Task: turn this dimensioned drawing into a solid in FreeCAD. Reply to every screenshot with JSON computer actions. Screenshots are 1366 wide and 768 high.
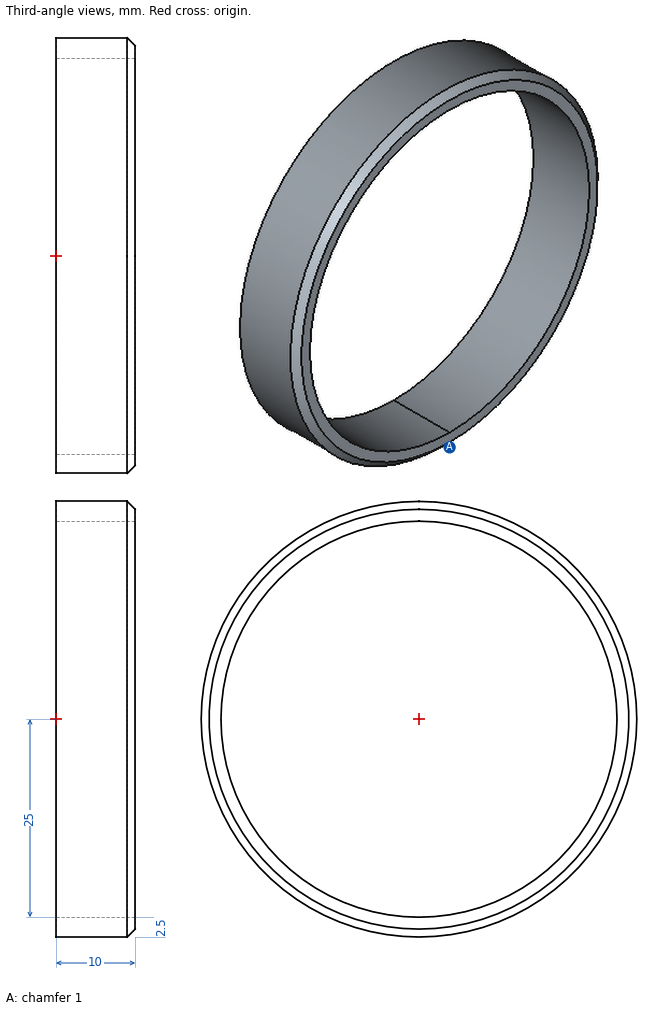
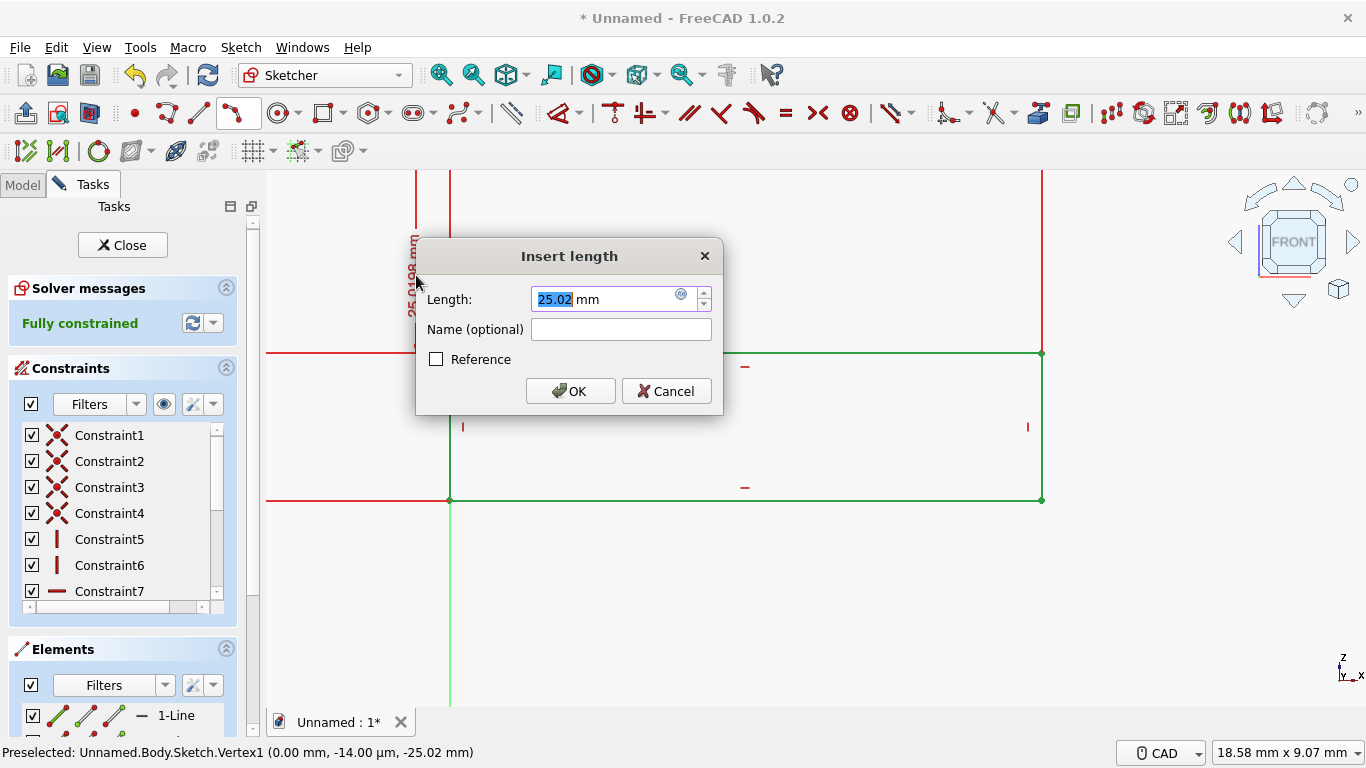
{"action": "type", "text": "25"}
{"action": "key", "text": "Return"}
{"action": "key", "text": "Escape"}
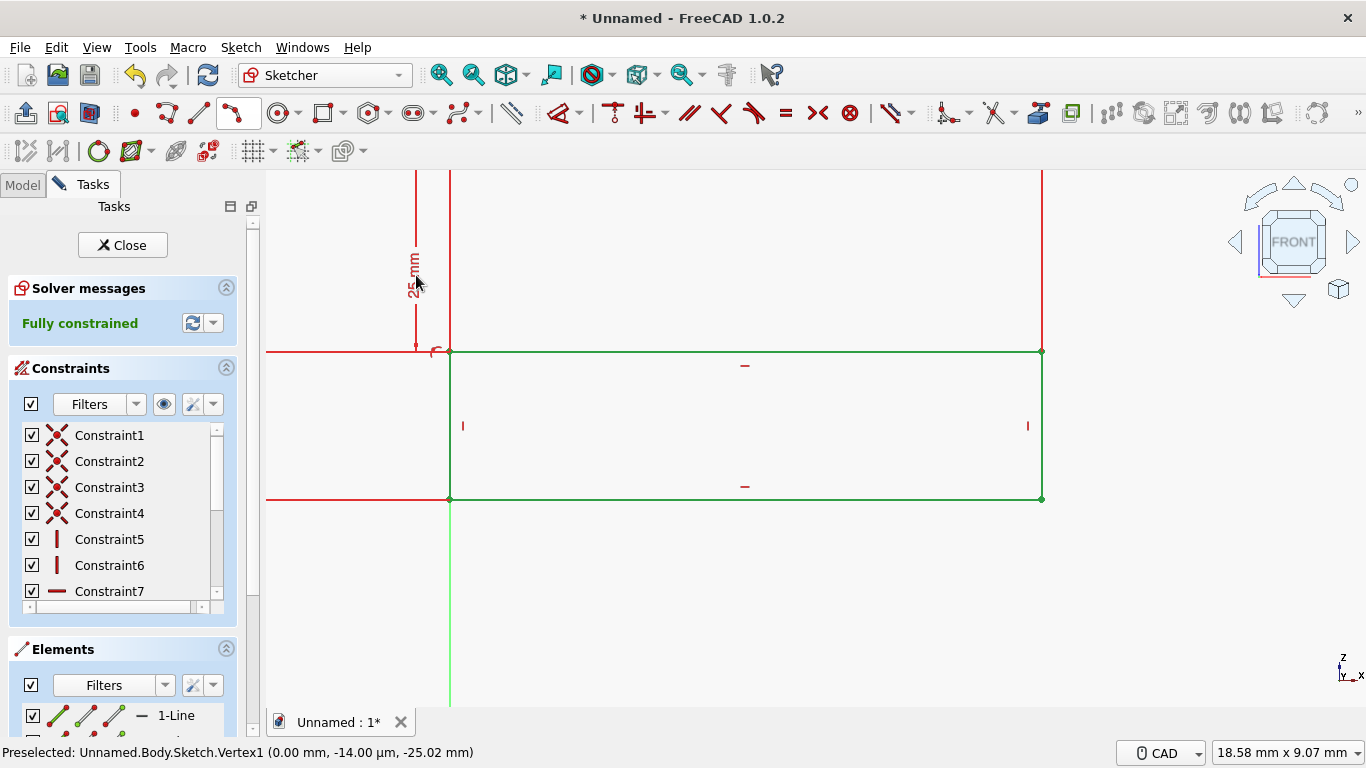
{"action": "left_click", "coordinate": [123, 245]}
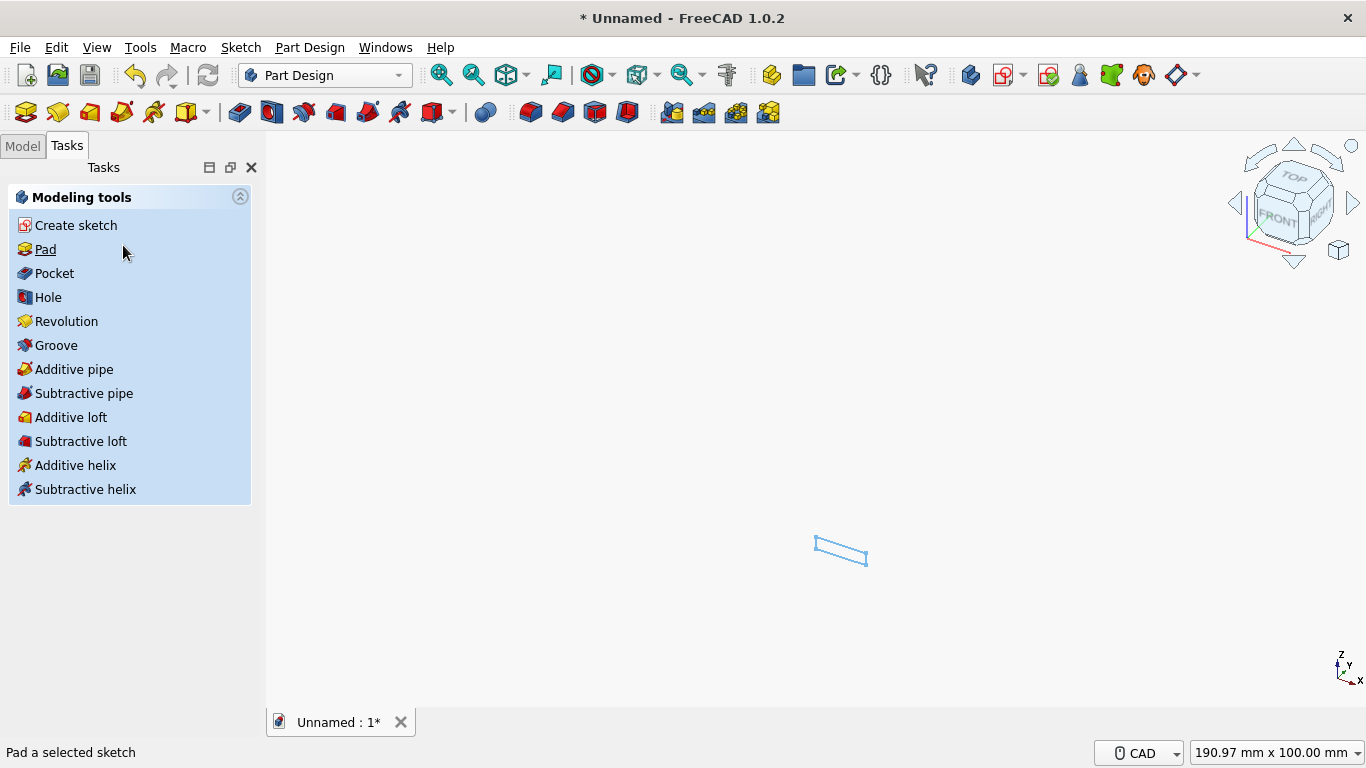
{"action": "left_click", "coordinate": [58, 112]}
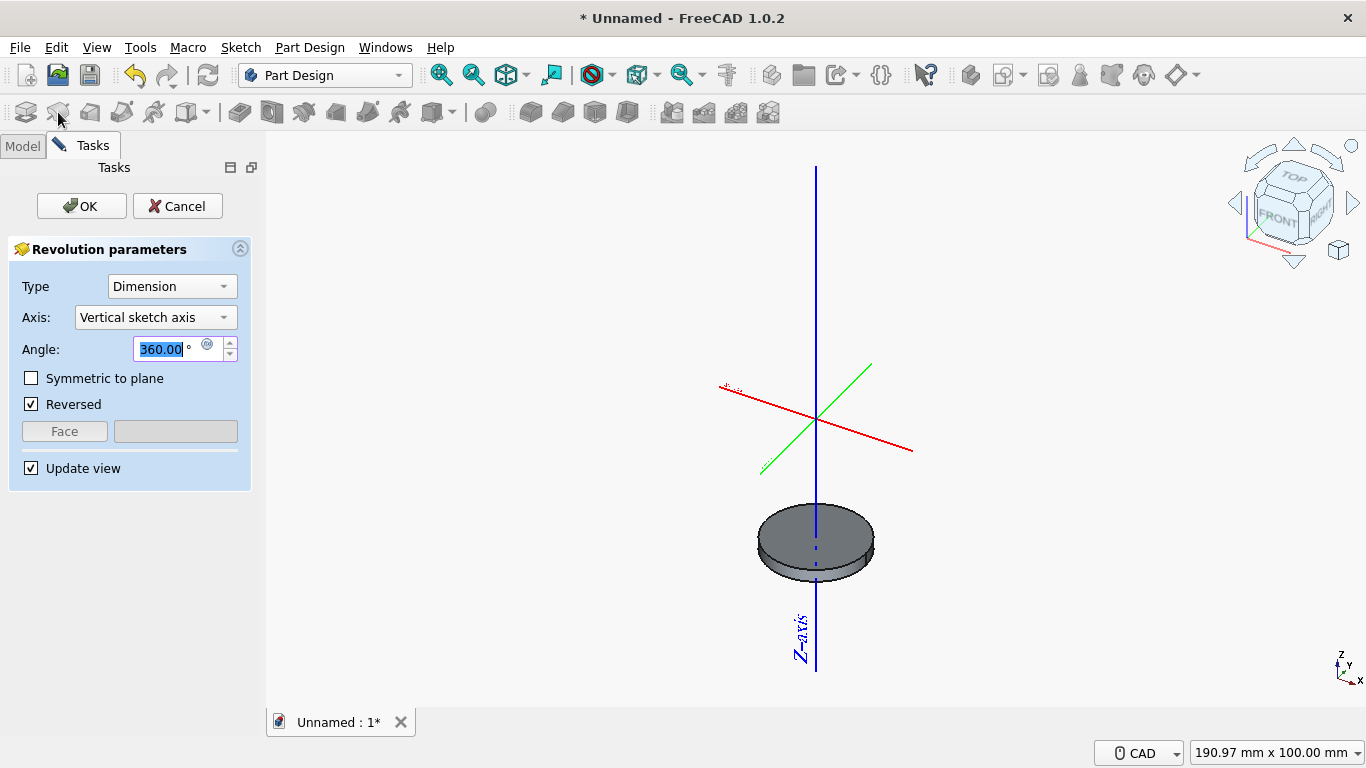
{"action": "left_click", "coordinate": [156, 318]}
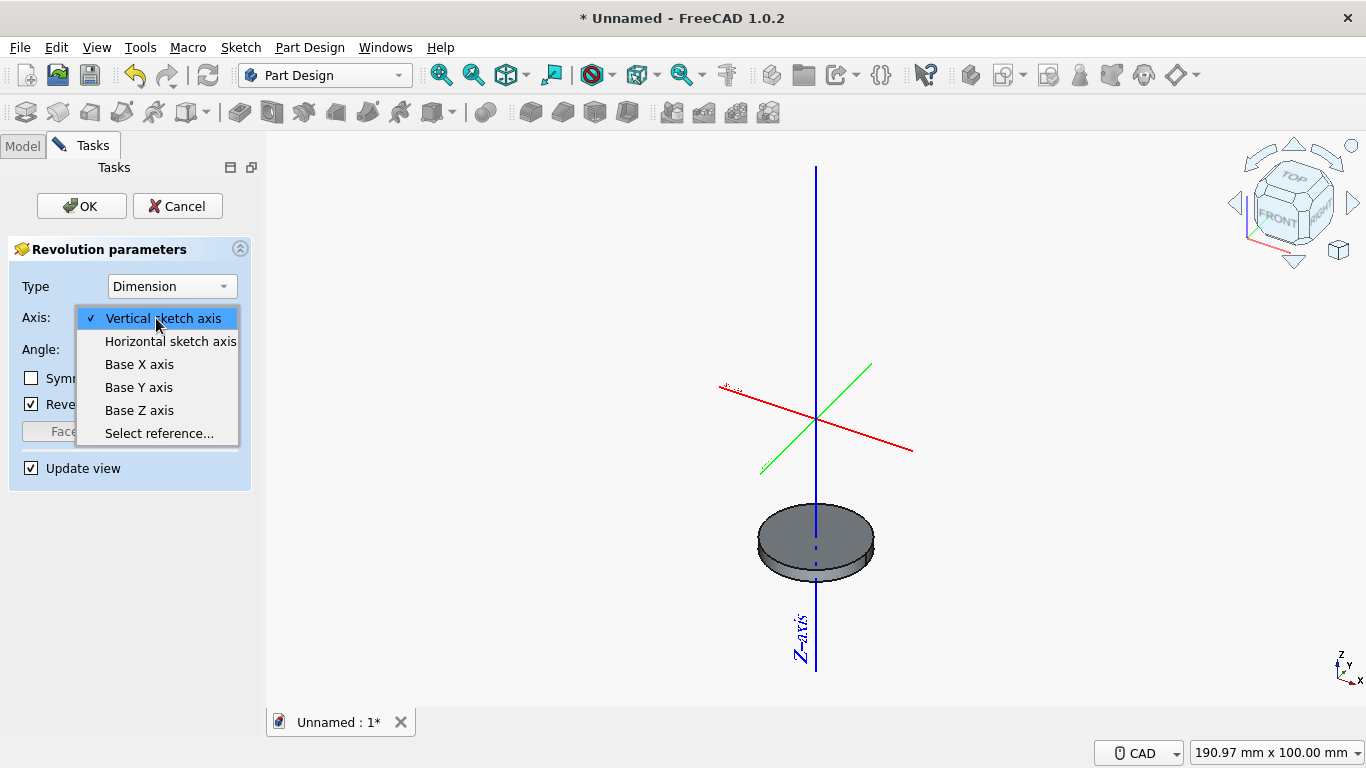
{"action": "left_click", "coordinate": [156, 342]}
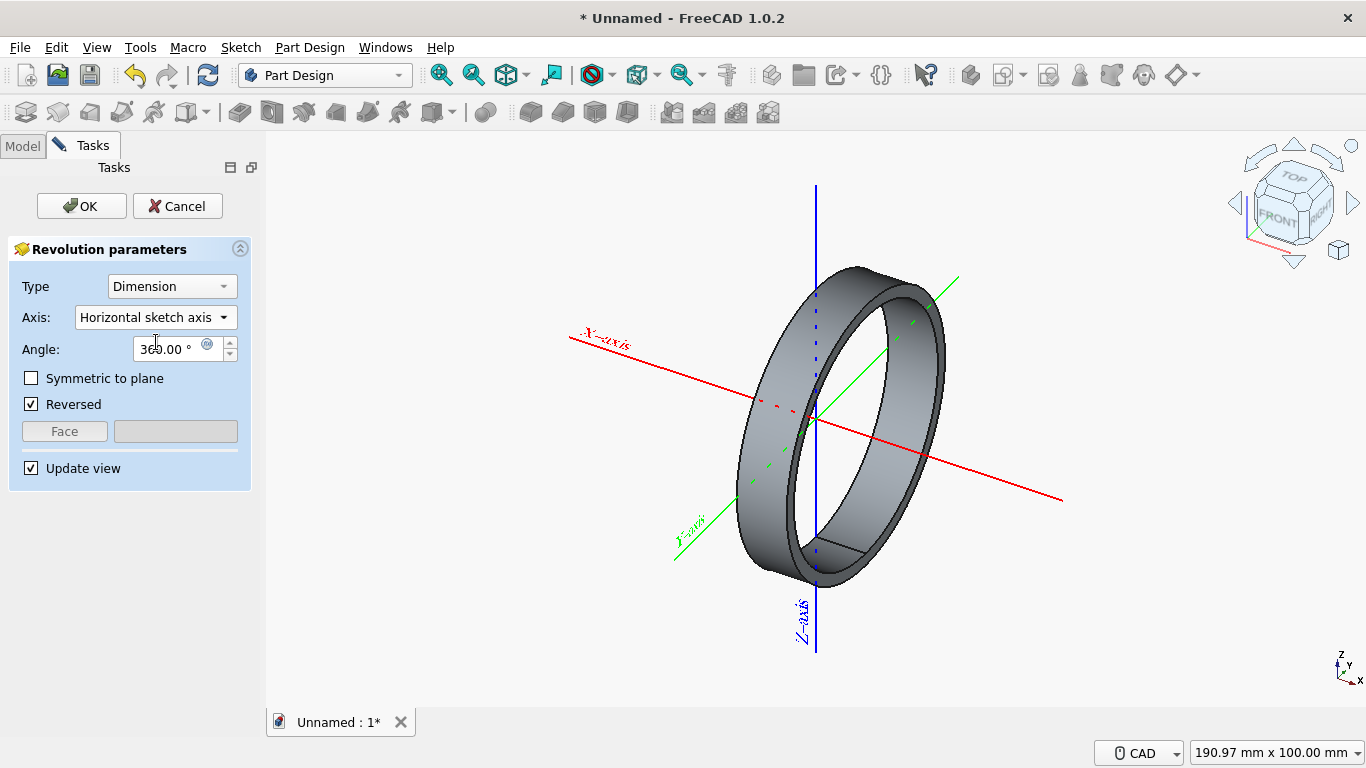
{"action": "left_click", "coordinate": [82, 206]}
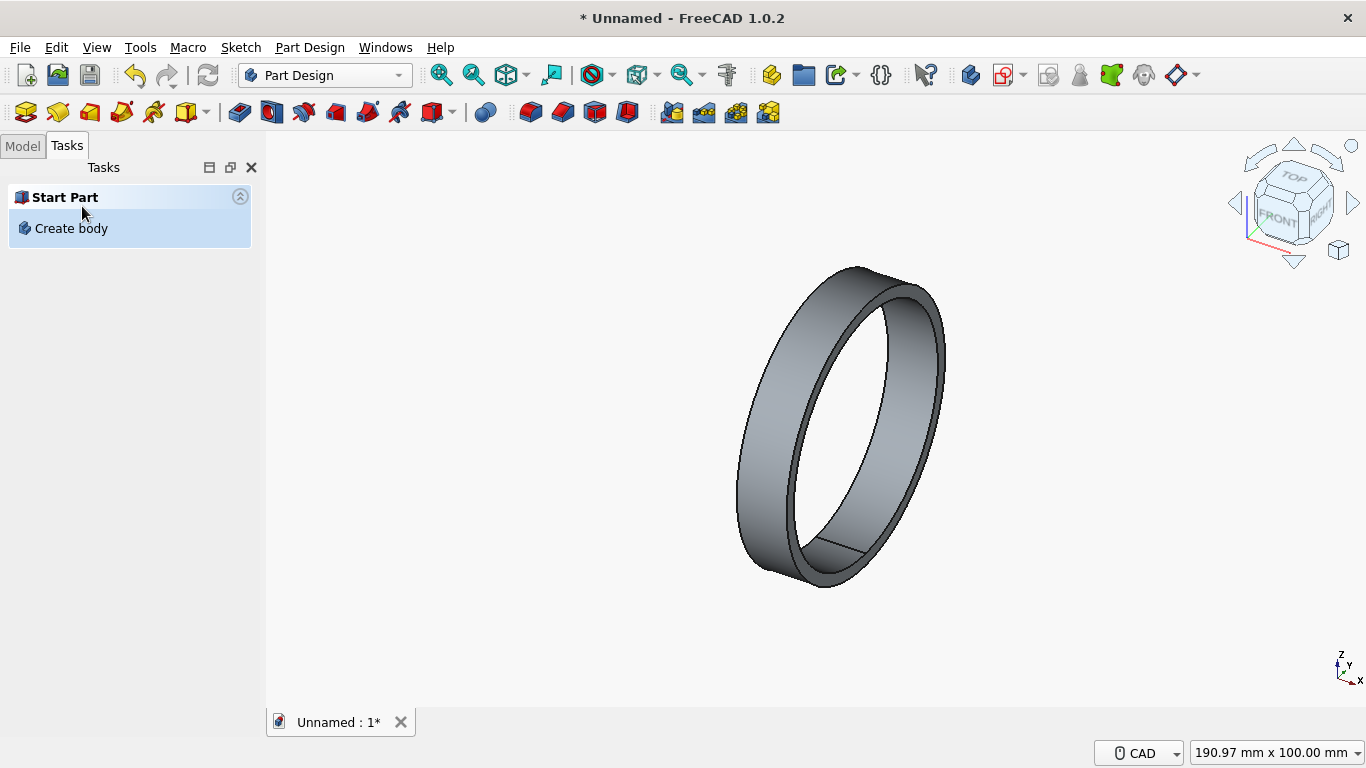
{"action": "left_click", "coordinate": [866, 305]}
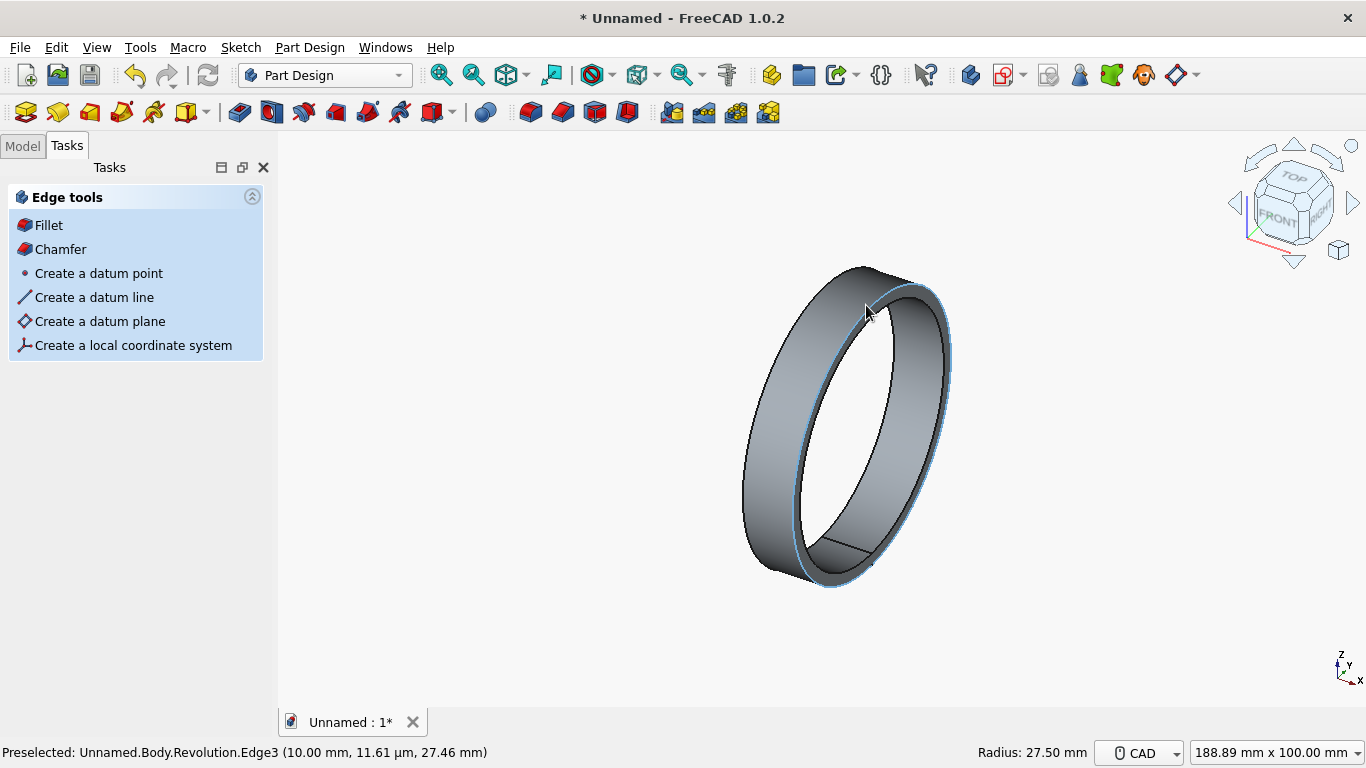
{"action": "left_click", "coordinate": [564, 112]}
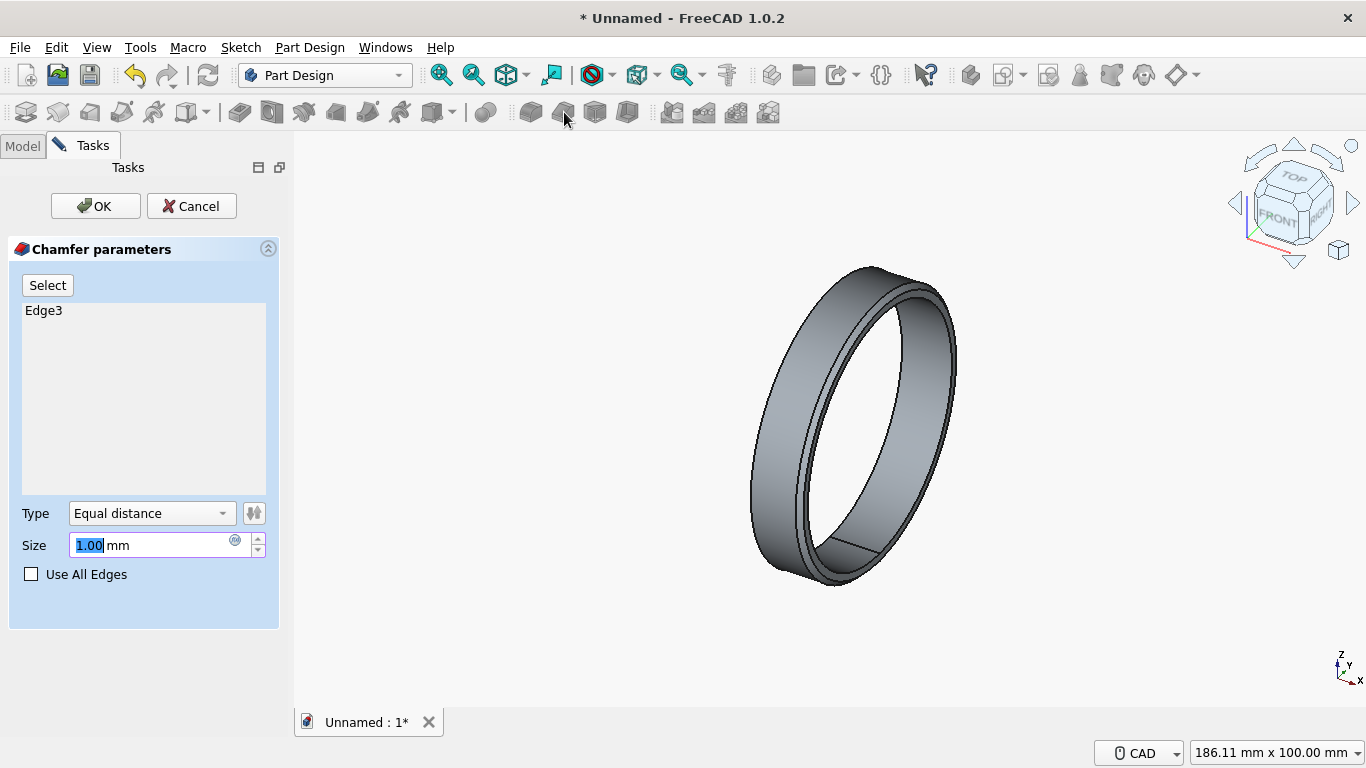
{"action": "type", "text": "1"}
{"action": "key", "text": "Tab"}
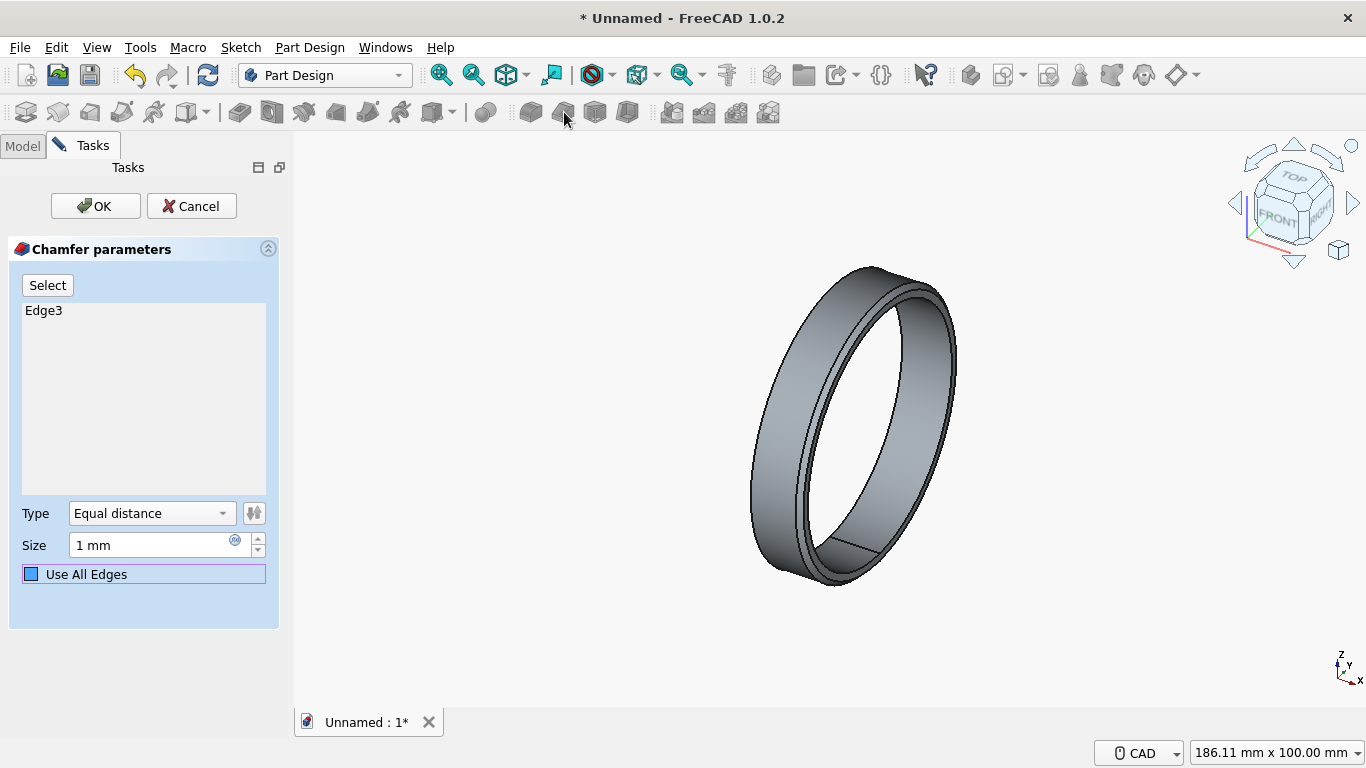
{"action": "left_click", "coordinate": [96, 206]}